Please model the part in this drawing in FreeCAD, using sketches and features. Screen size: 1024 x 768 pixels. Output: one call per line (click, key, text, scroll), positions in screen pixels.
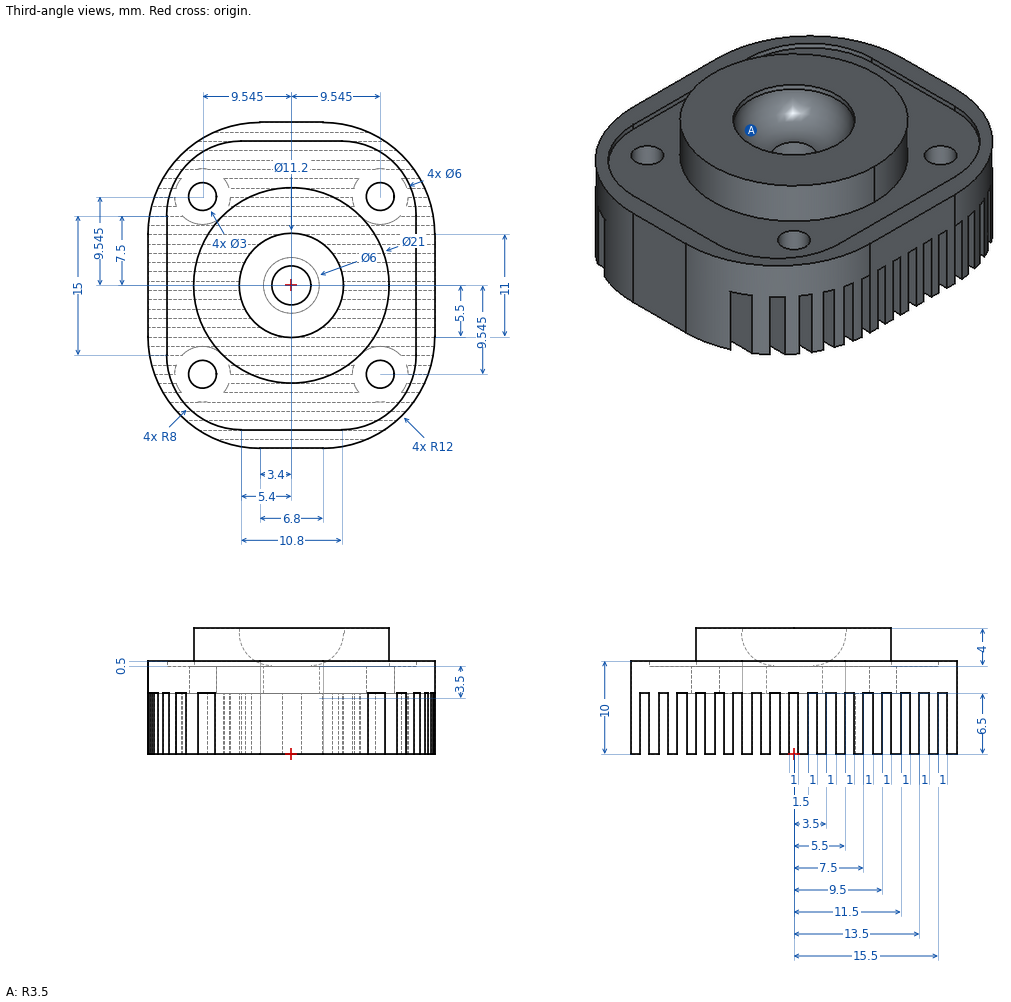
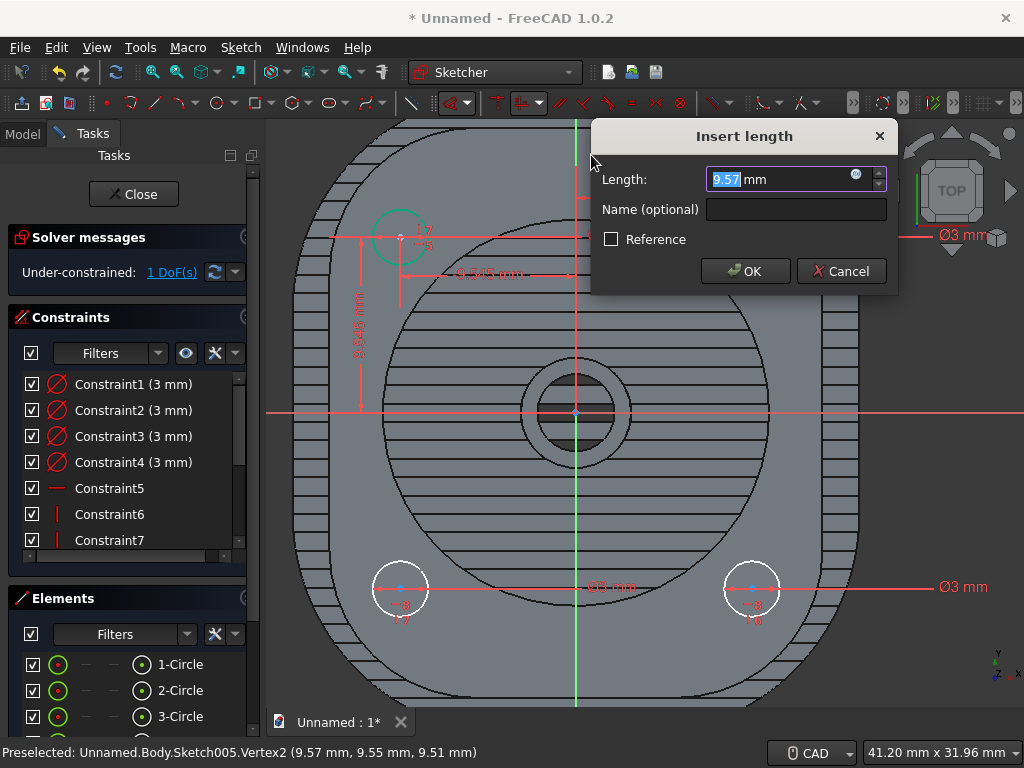
text(9.545)
key(Return)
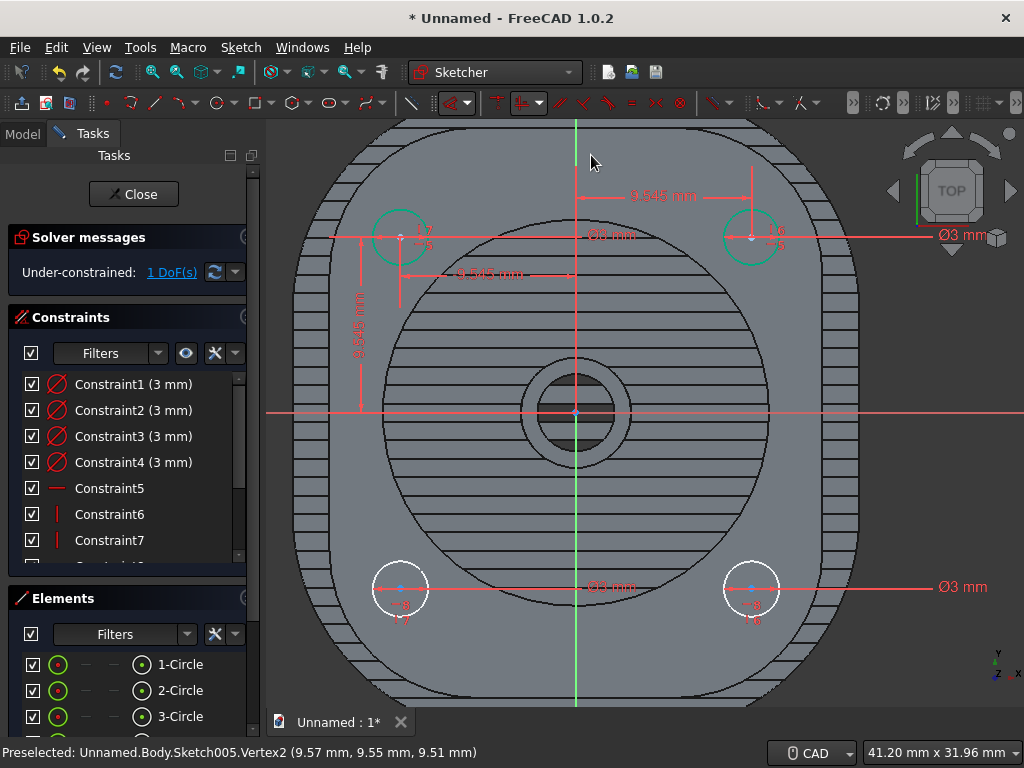
click(752, 589)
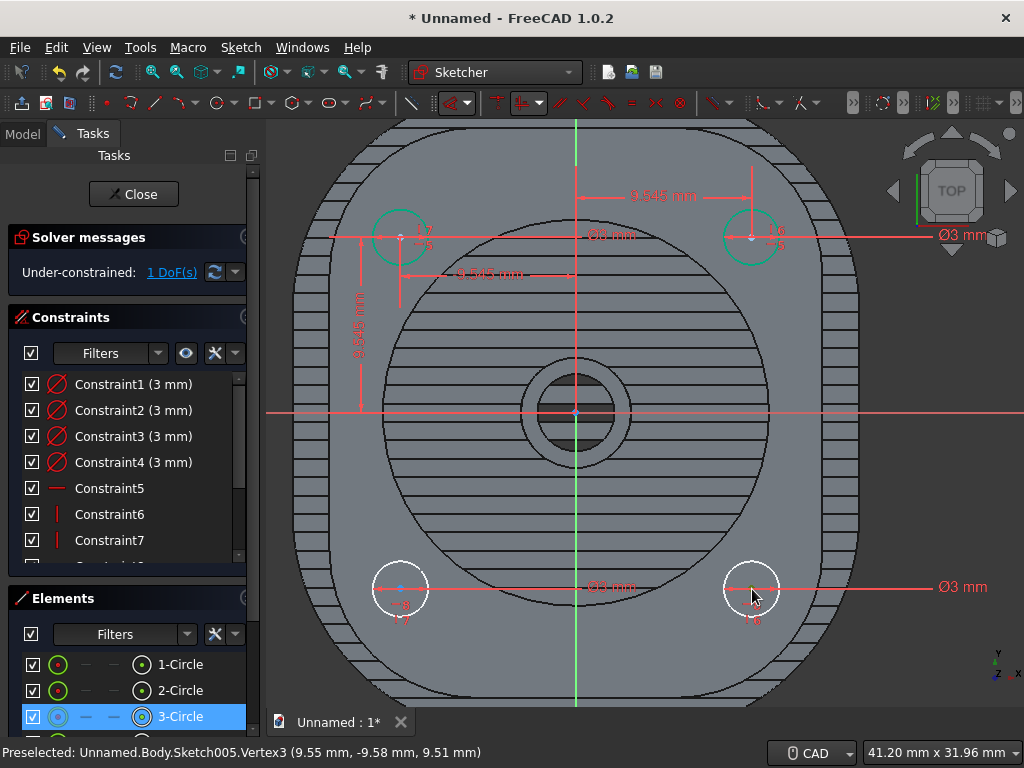
click(470, 104)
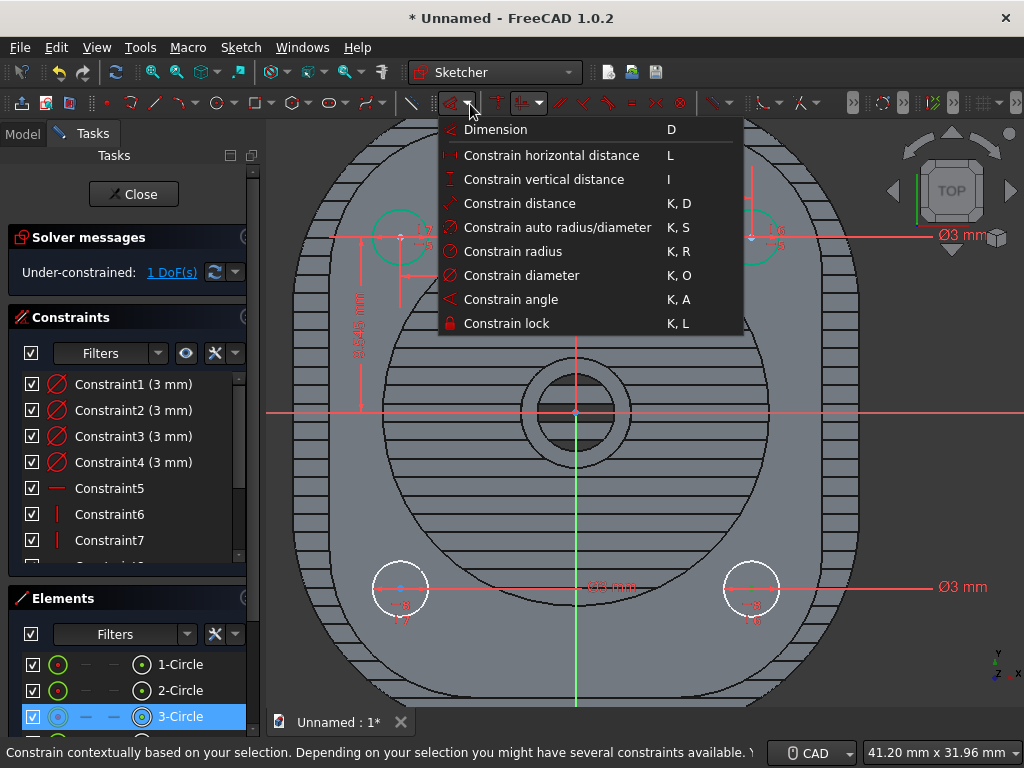
click(591, 179)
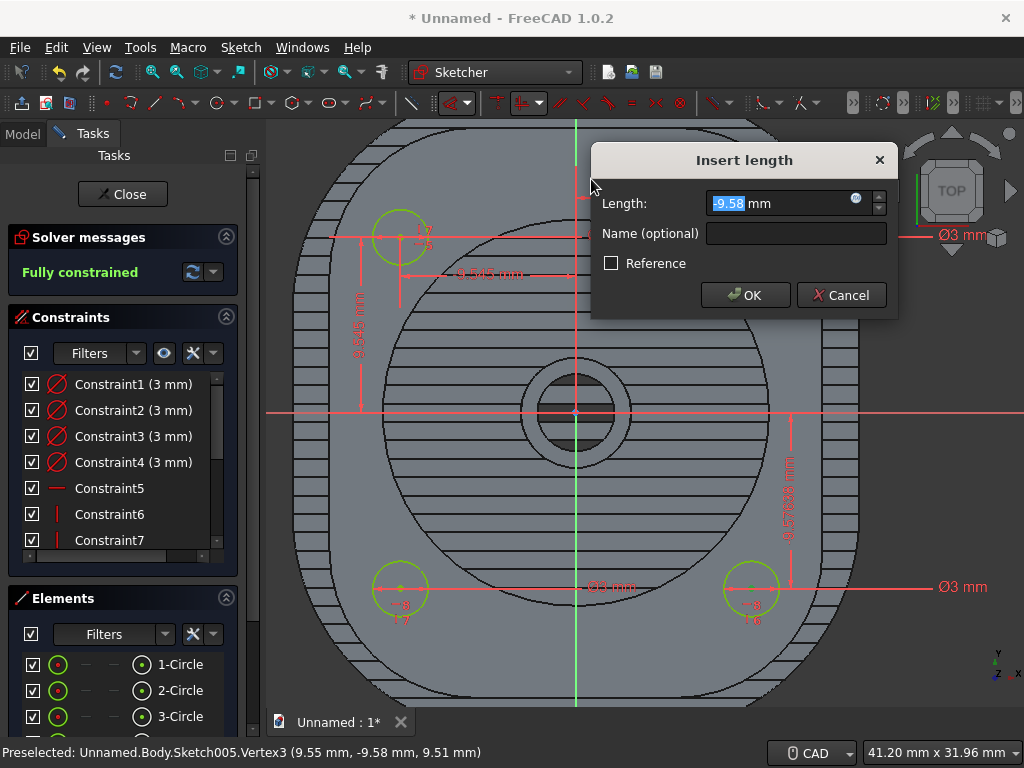
text(-9.545)
key(Return)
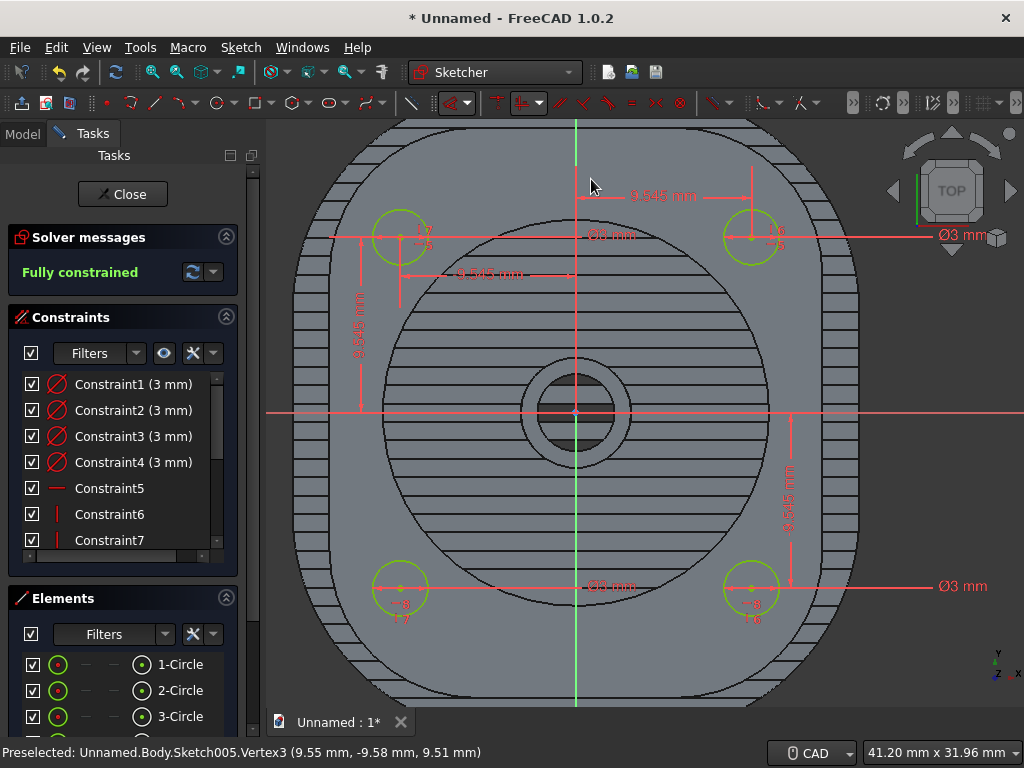
click(123, 194)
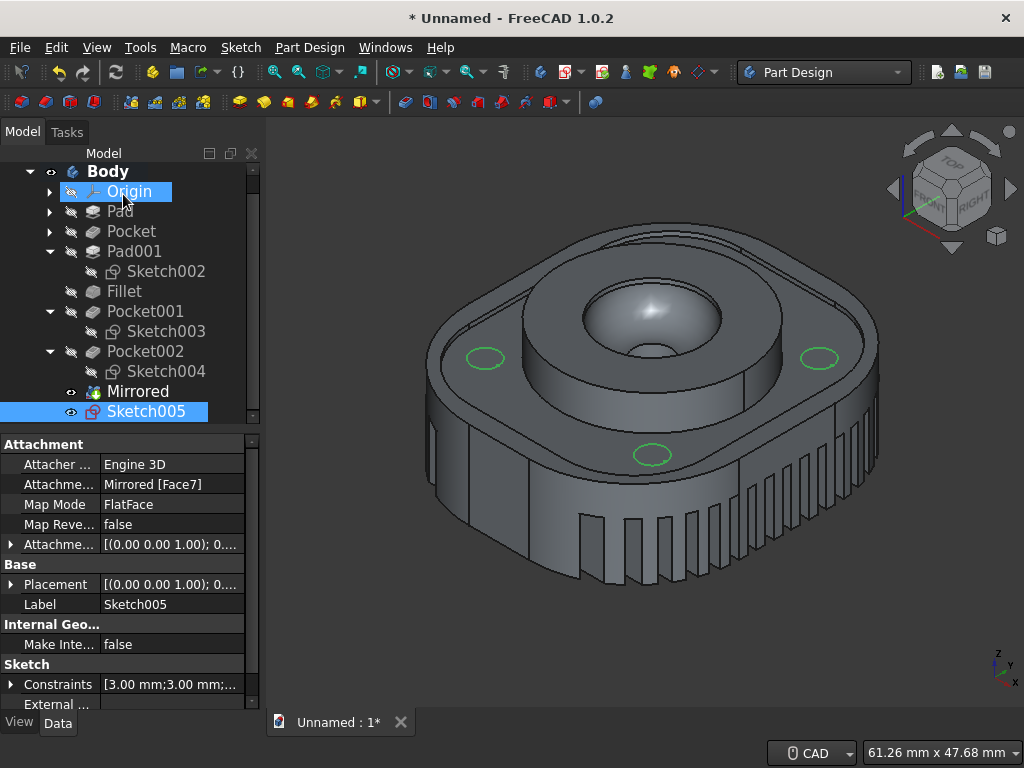
click(406, 102)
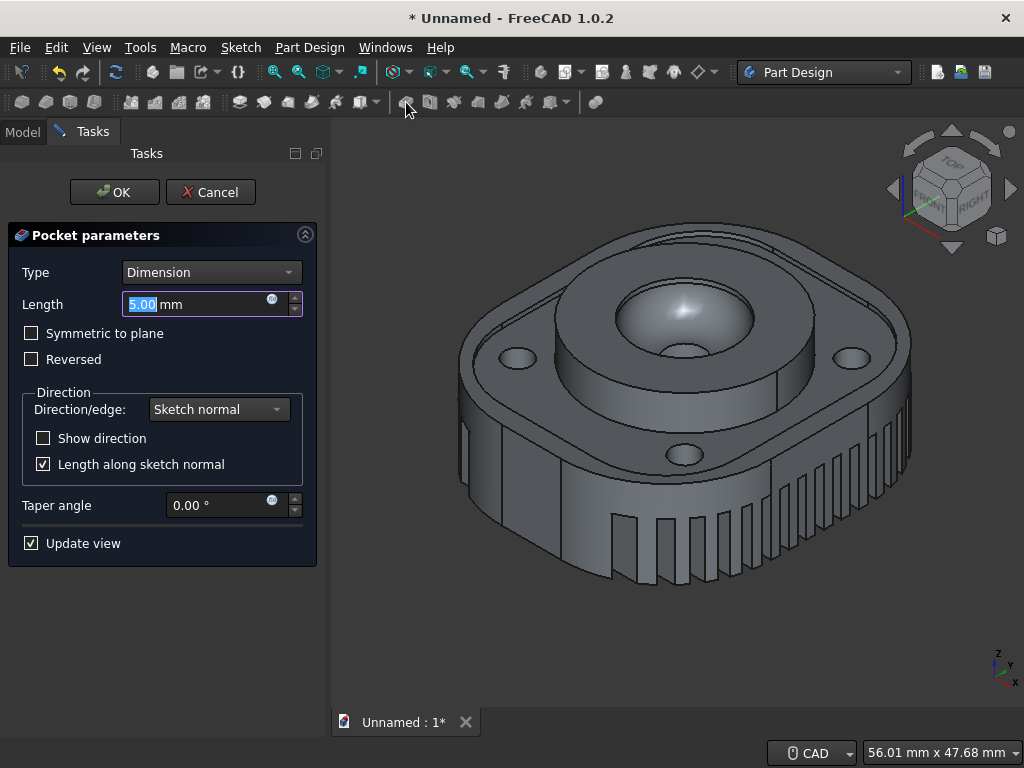
text(3.5)
key(Tab)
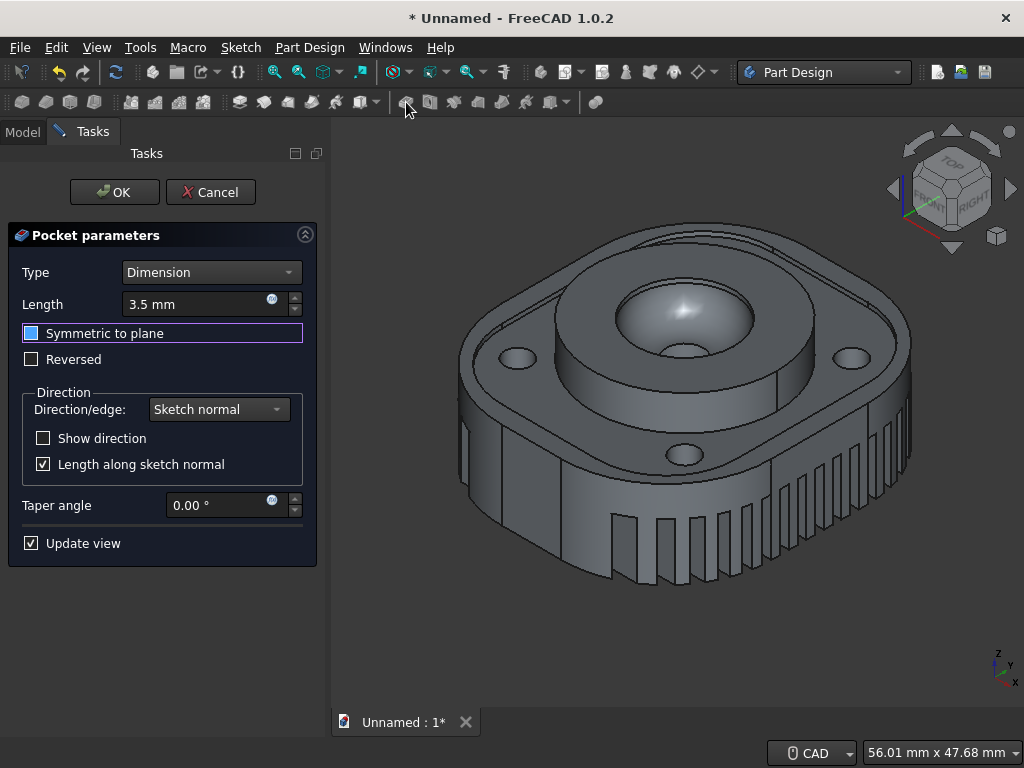
click(115, 192)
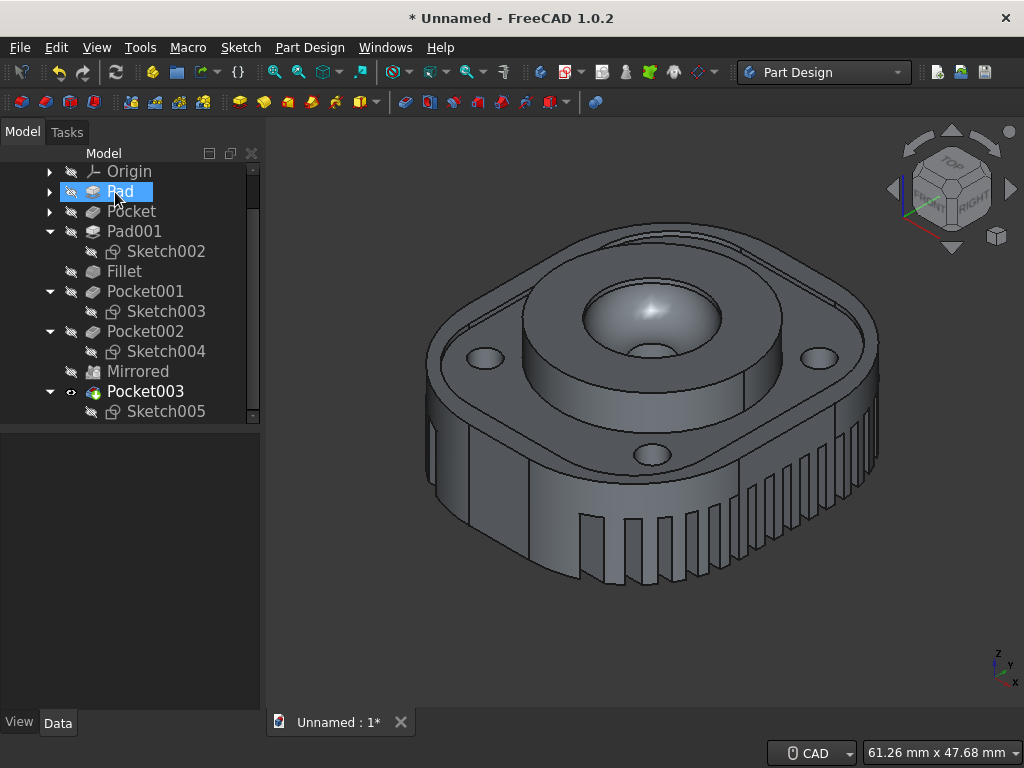
key(5)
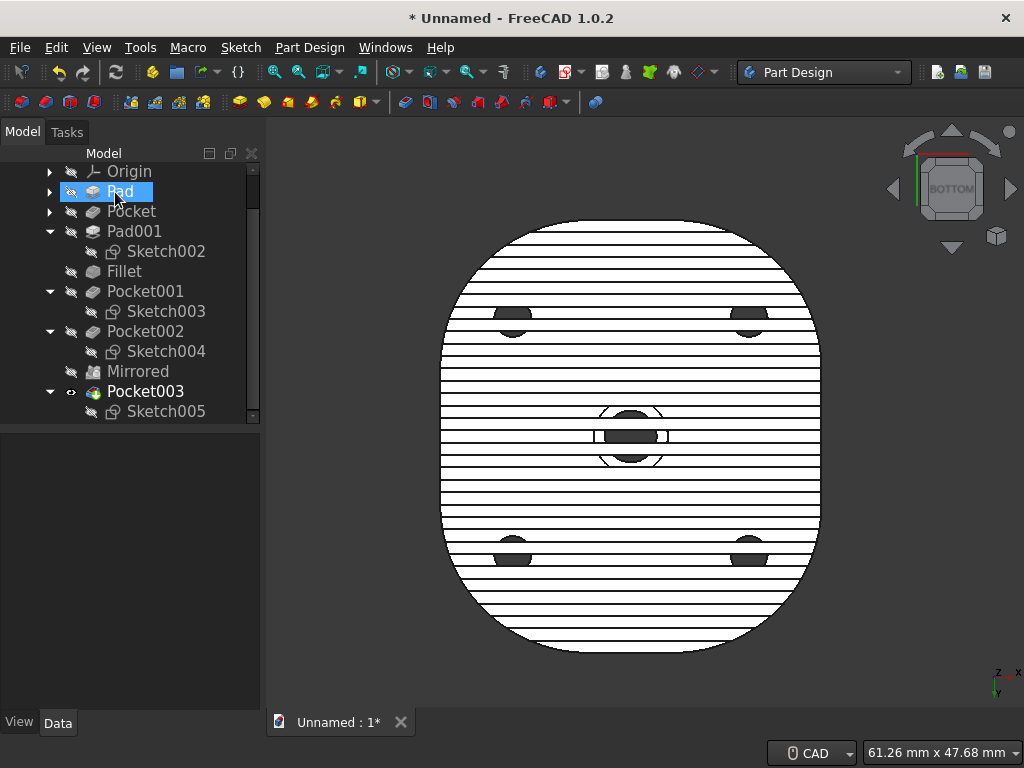
scroll(794, 485, up, 4)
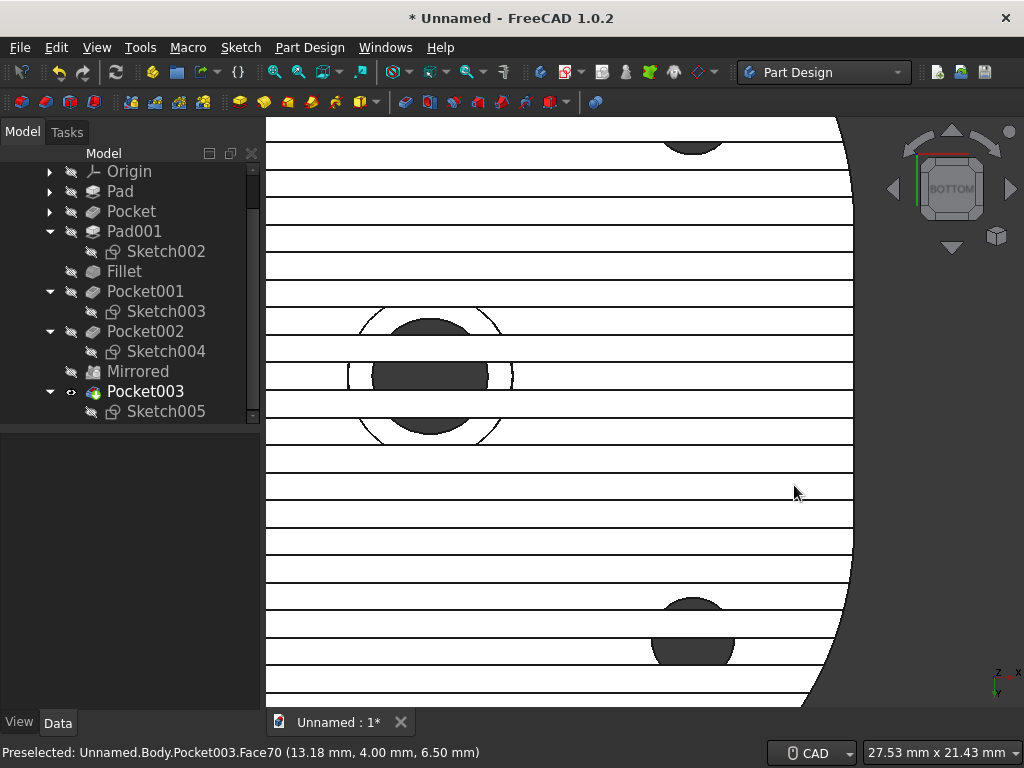
click(794, 485)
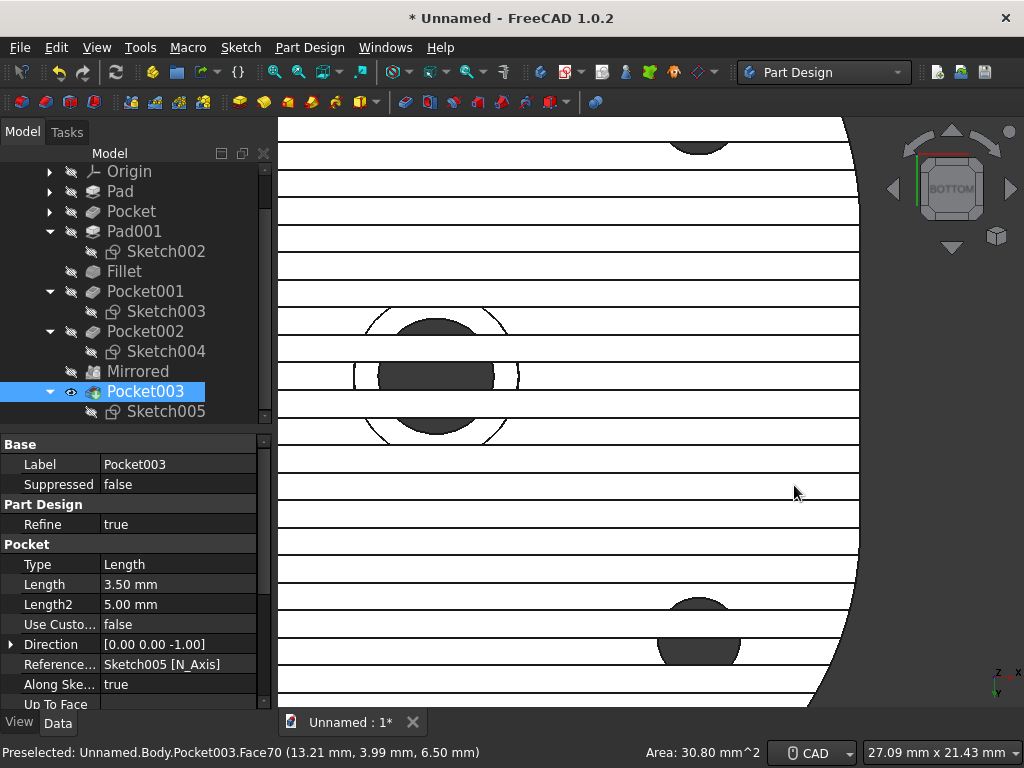
click(566, 72)